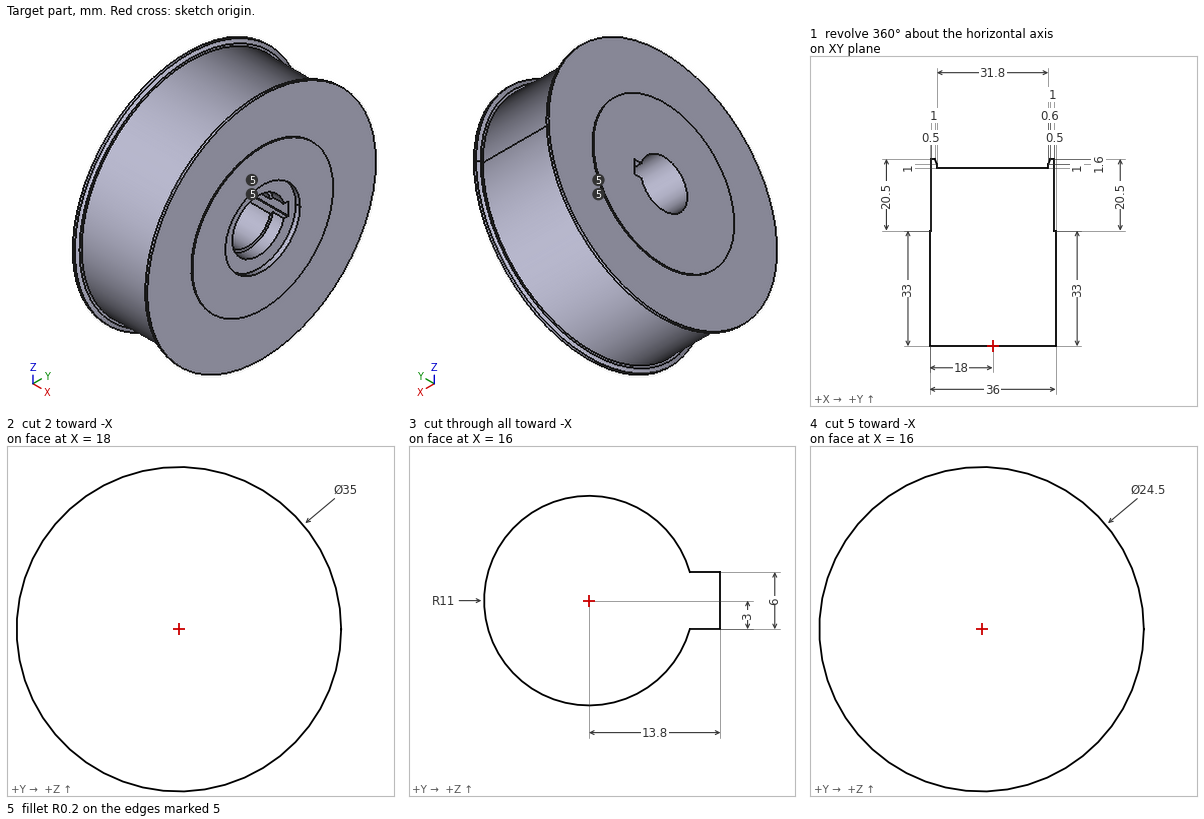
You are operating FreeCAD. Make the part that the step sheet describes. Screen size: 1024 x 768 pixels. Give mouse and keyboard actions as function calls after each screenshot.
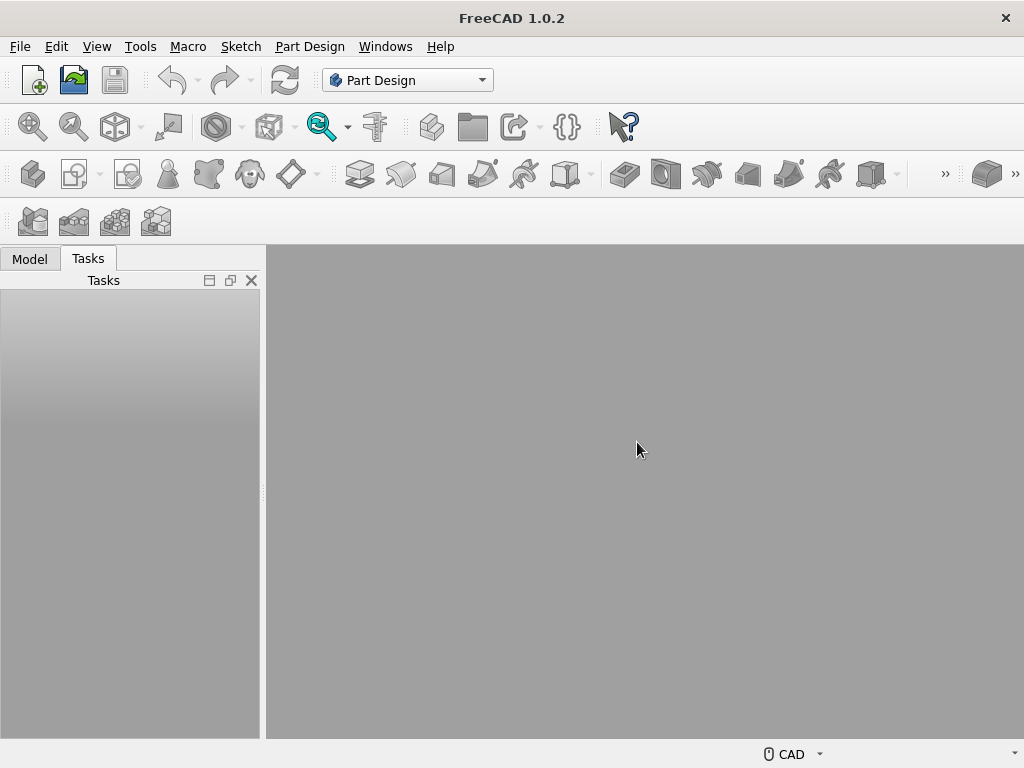
key(ctrl+n)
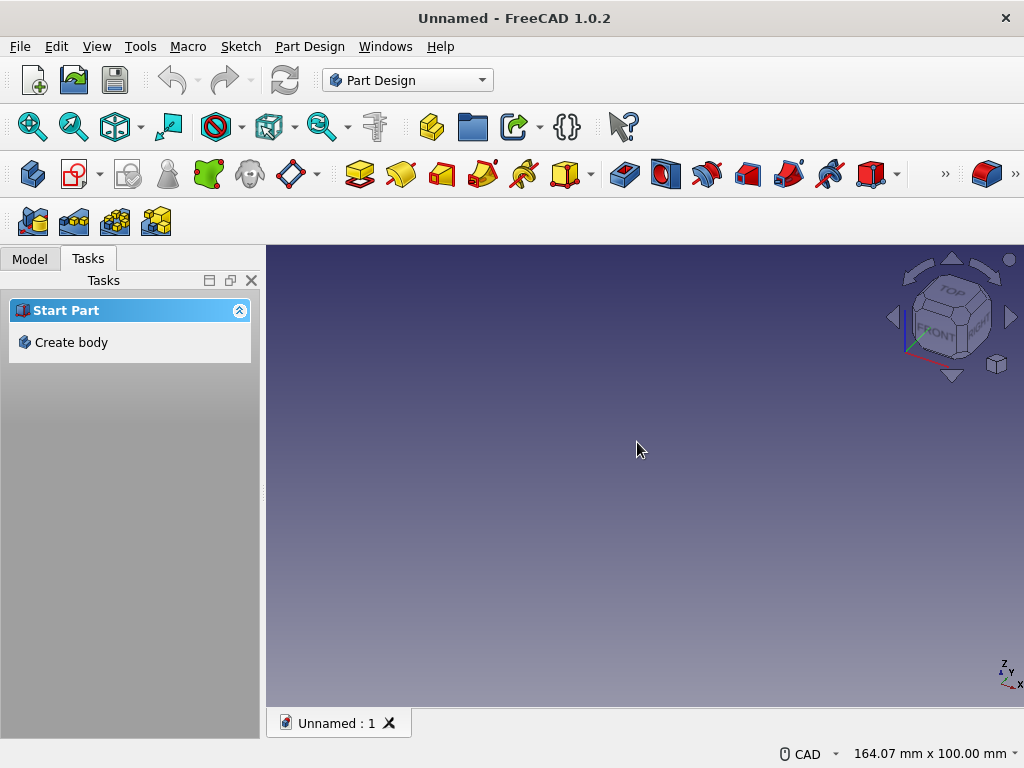
click(74, 174)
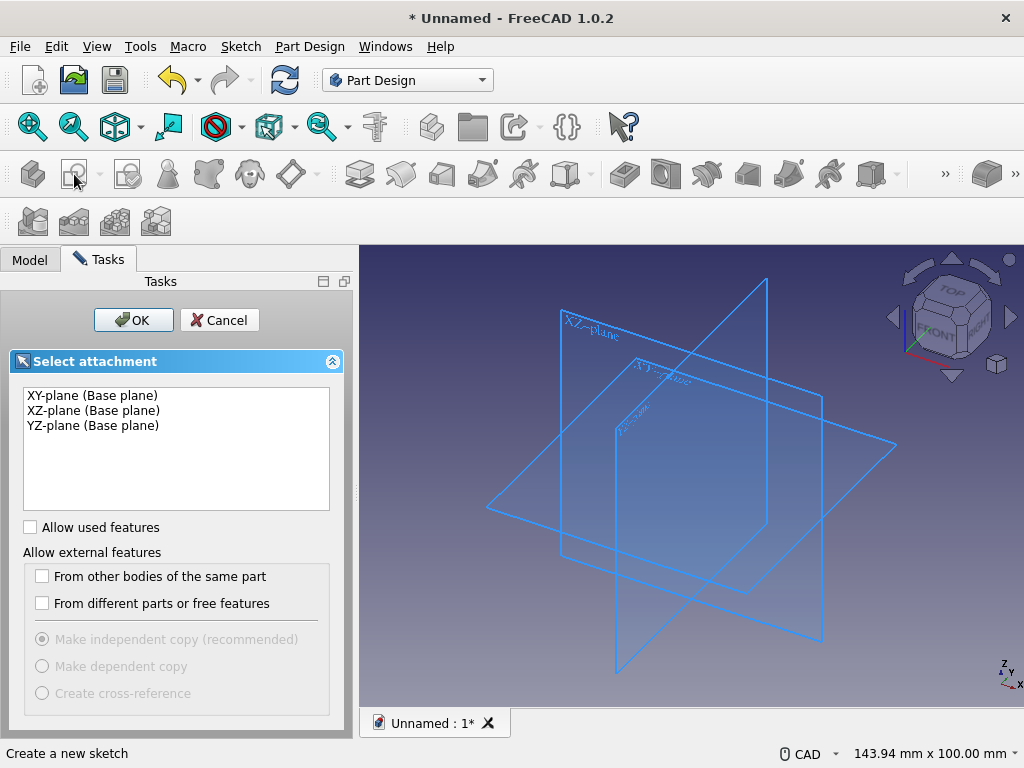
click(84, 396)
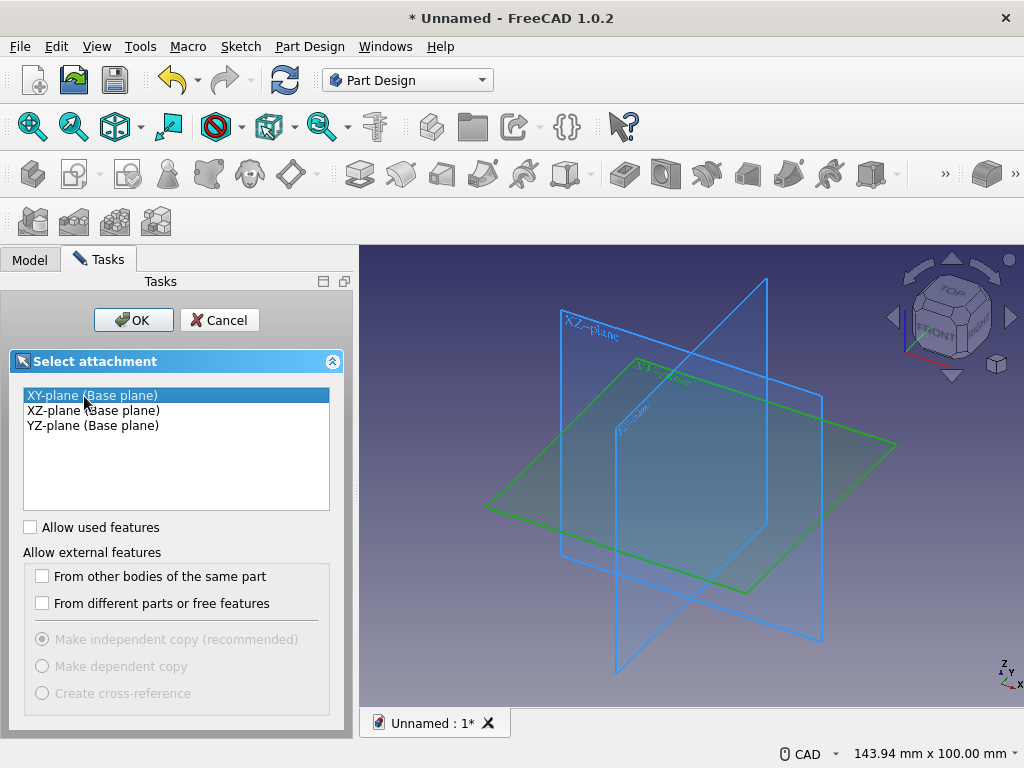
click(134, 320)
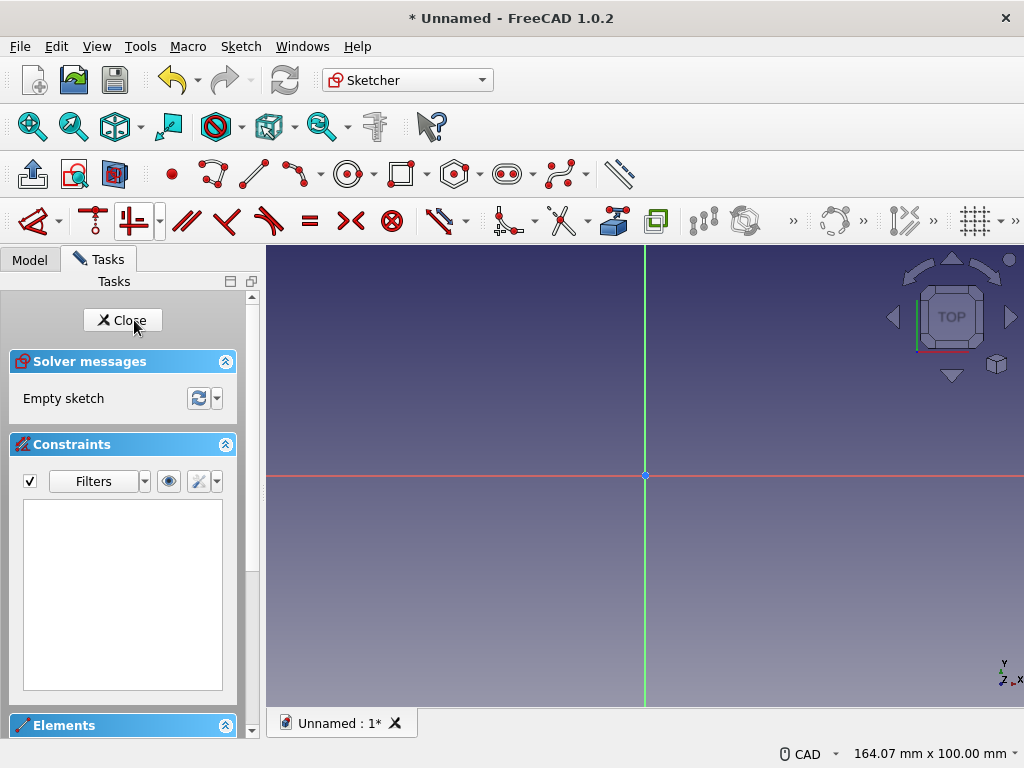
scroll(294, 679, down, 1)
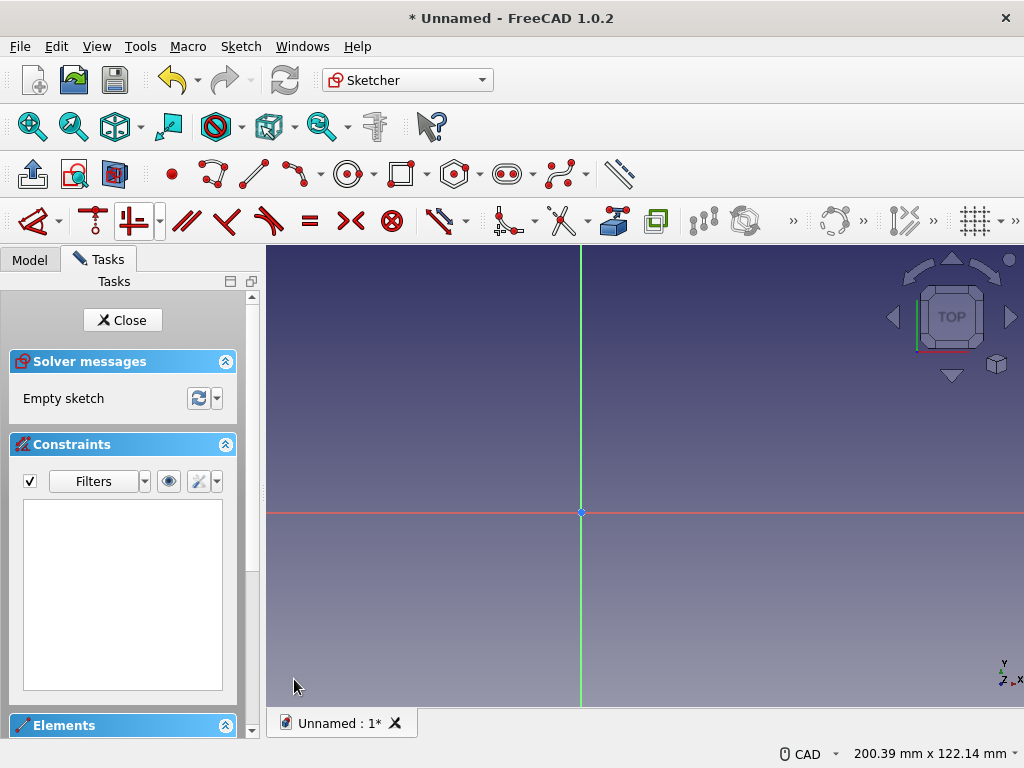
scroll(591, 281, up, 2)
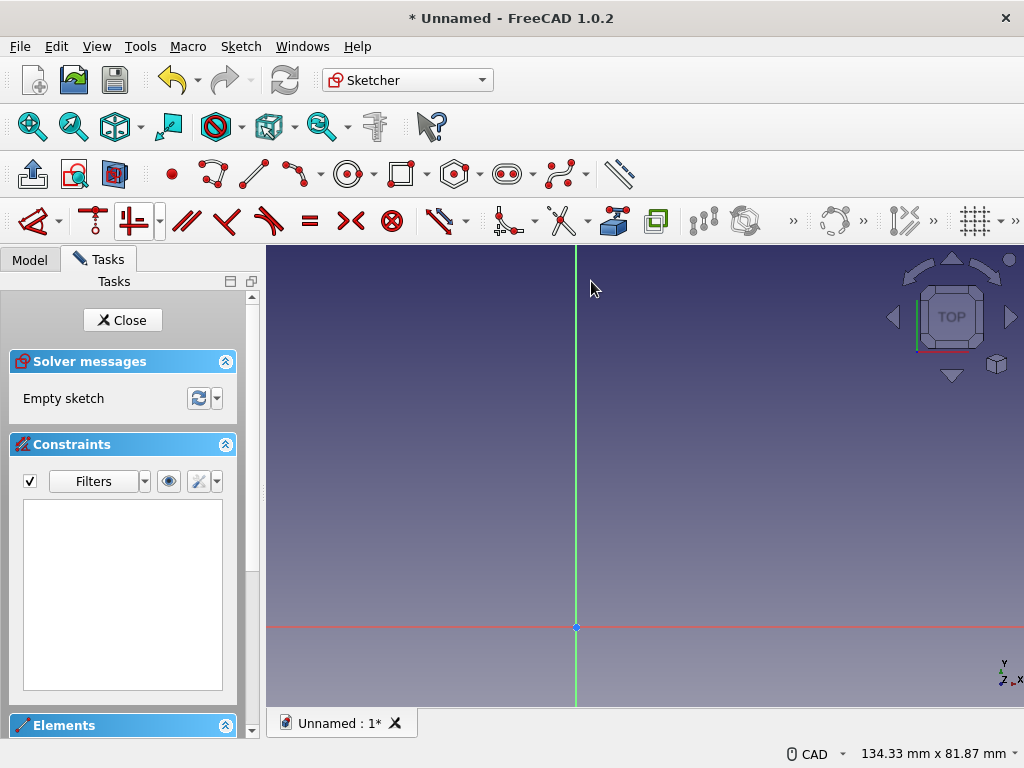
click(213, 174)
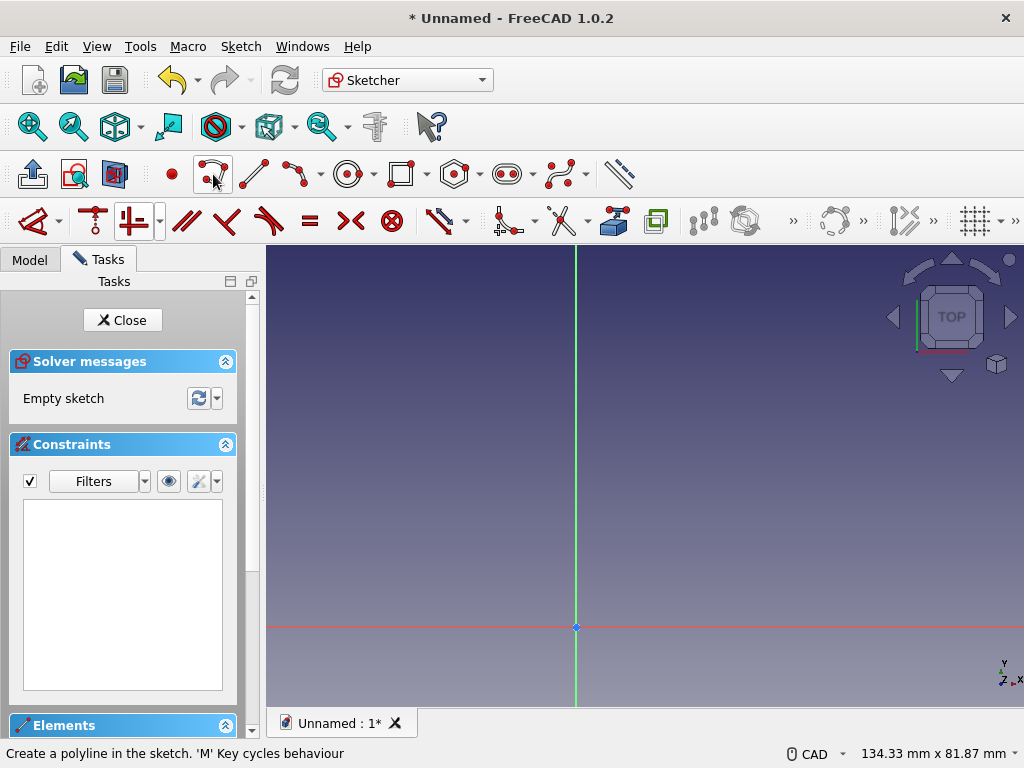
click(475, 627)
click(678, 618)
click(678, 441)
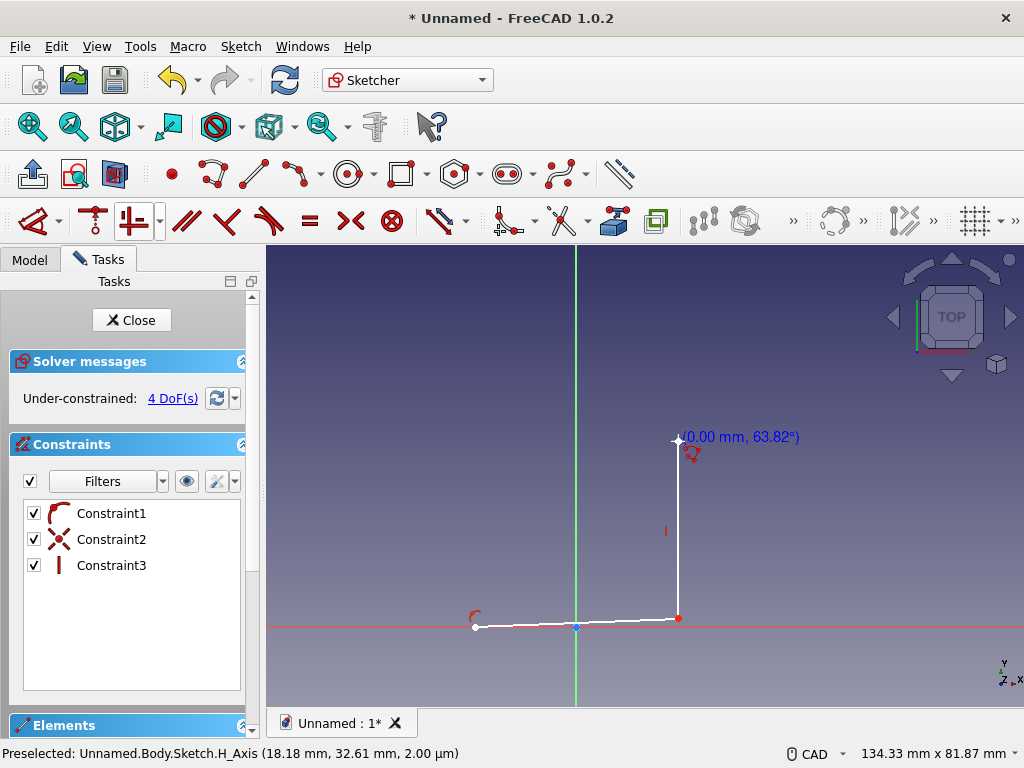
scroll(675, 441, up, 9)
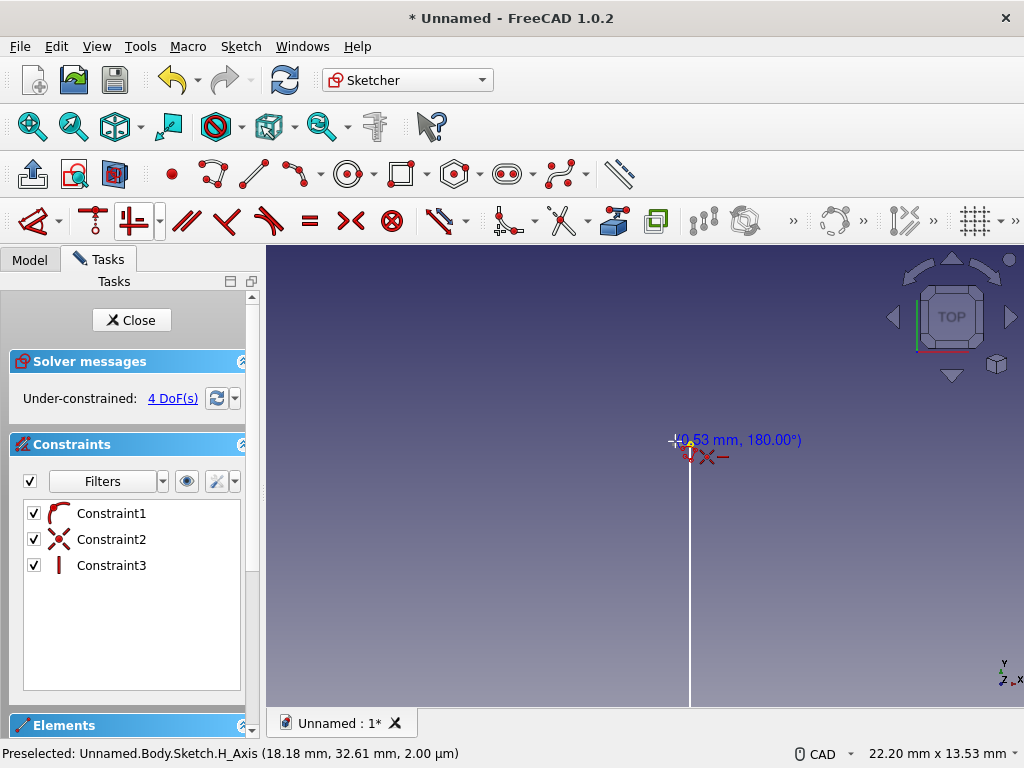
click(673, 439)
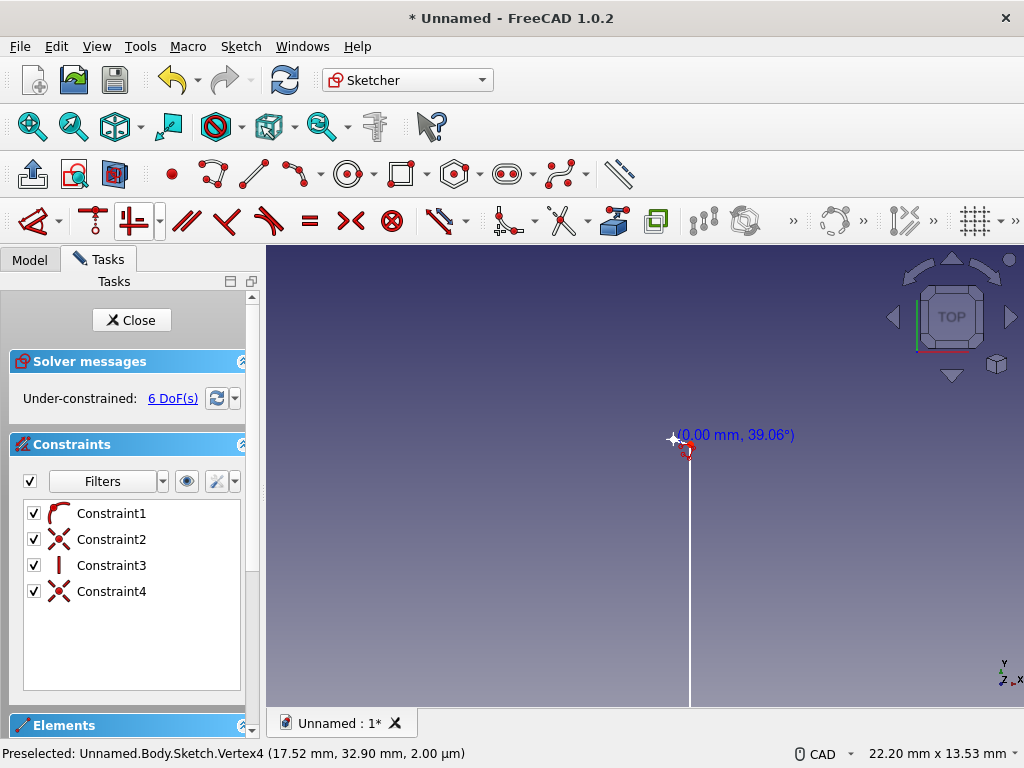
scroll(676, 441, down, 9)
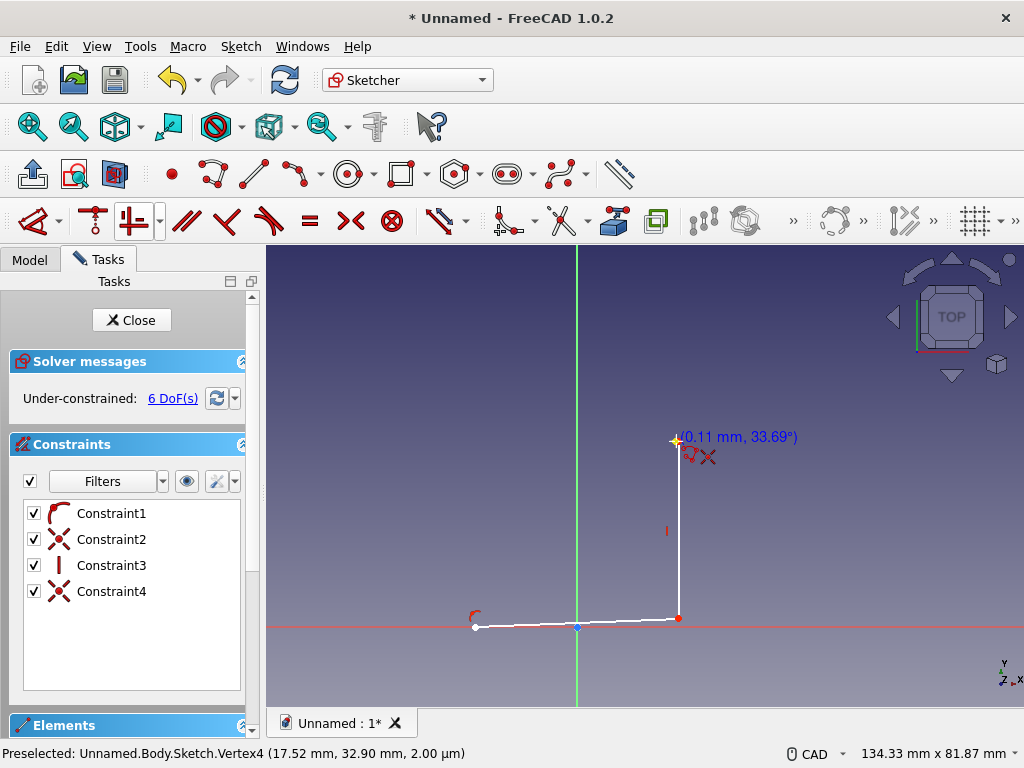
click(676, 325)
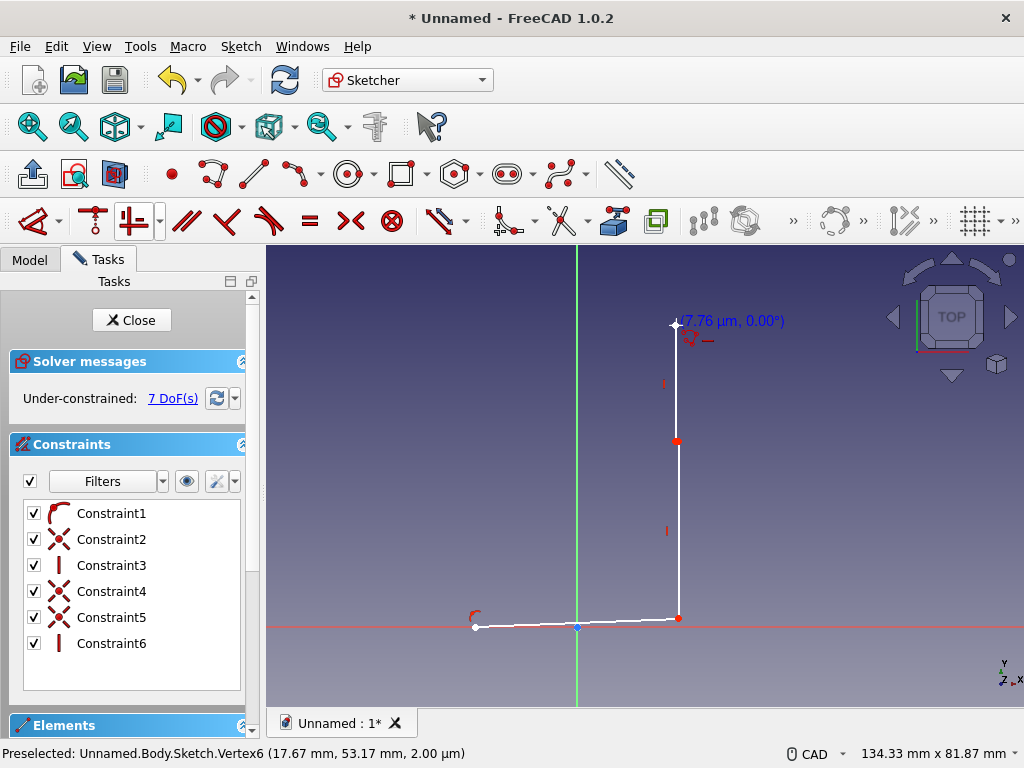
scroll(670, 325, up, 6)